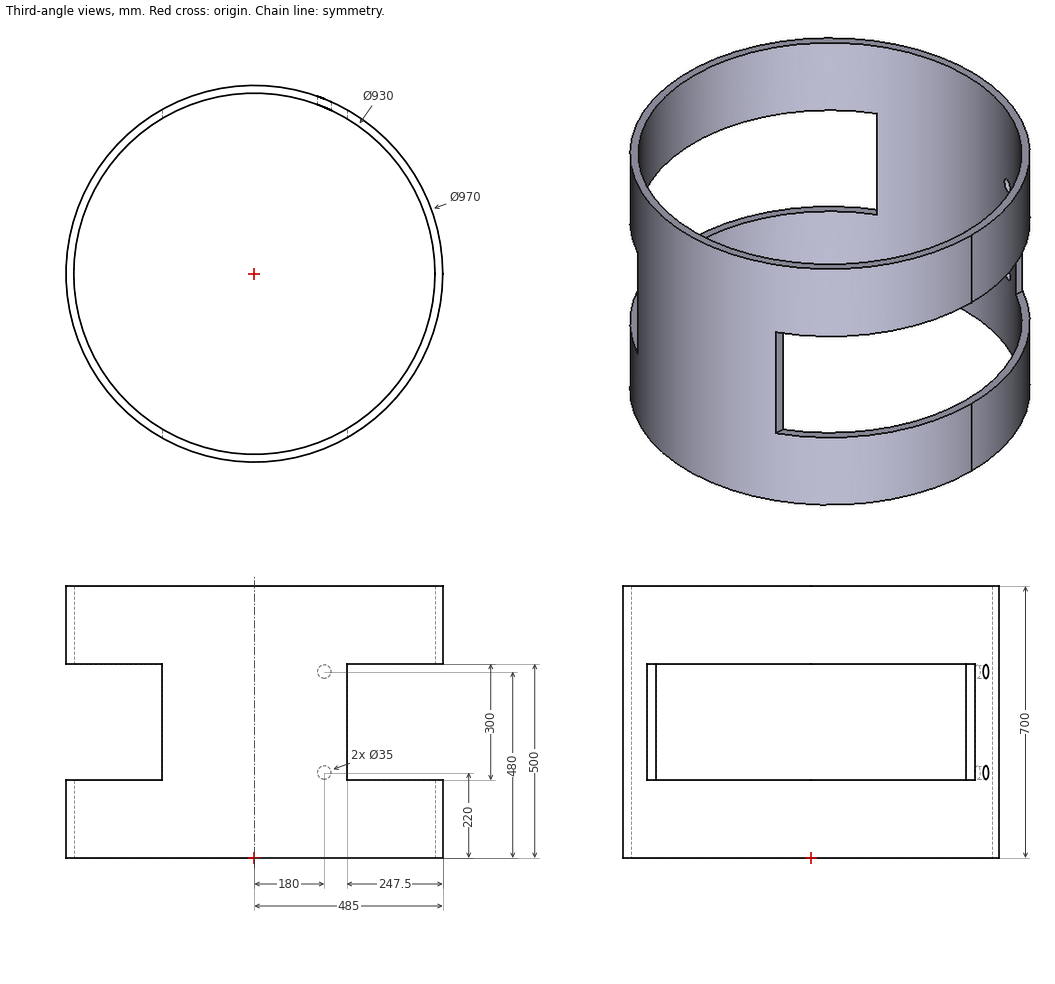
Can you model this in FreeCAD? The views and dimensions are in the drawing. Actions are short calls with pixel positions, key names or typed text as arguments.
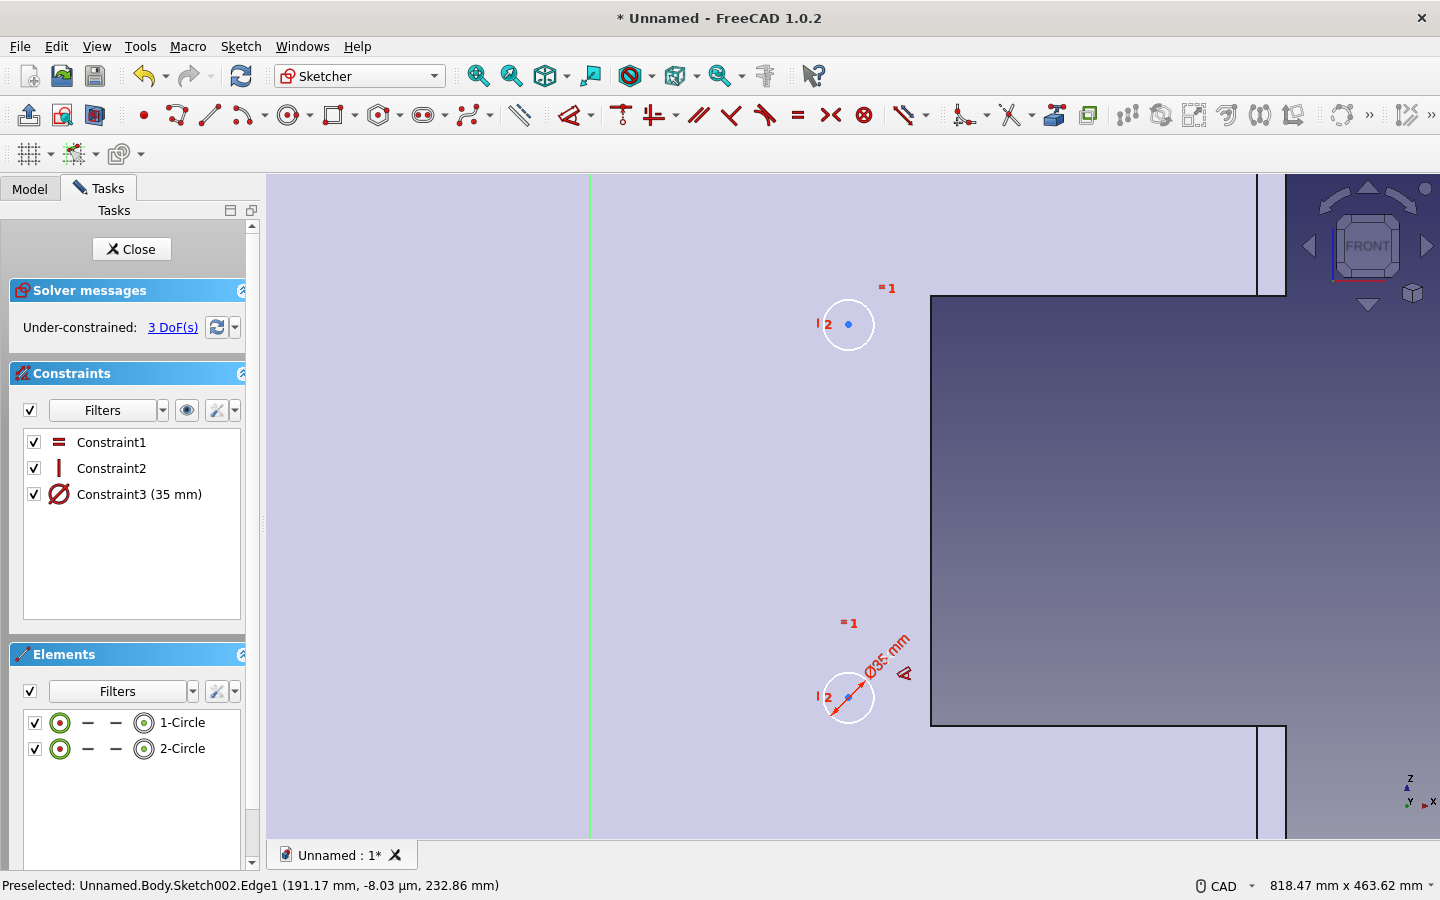
click(849, 698)
click(719, 664)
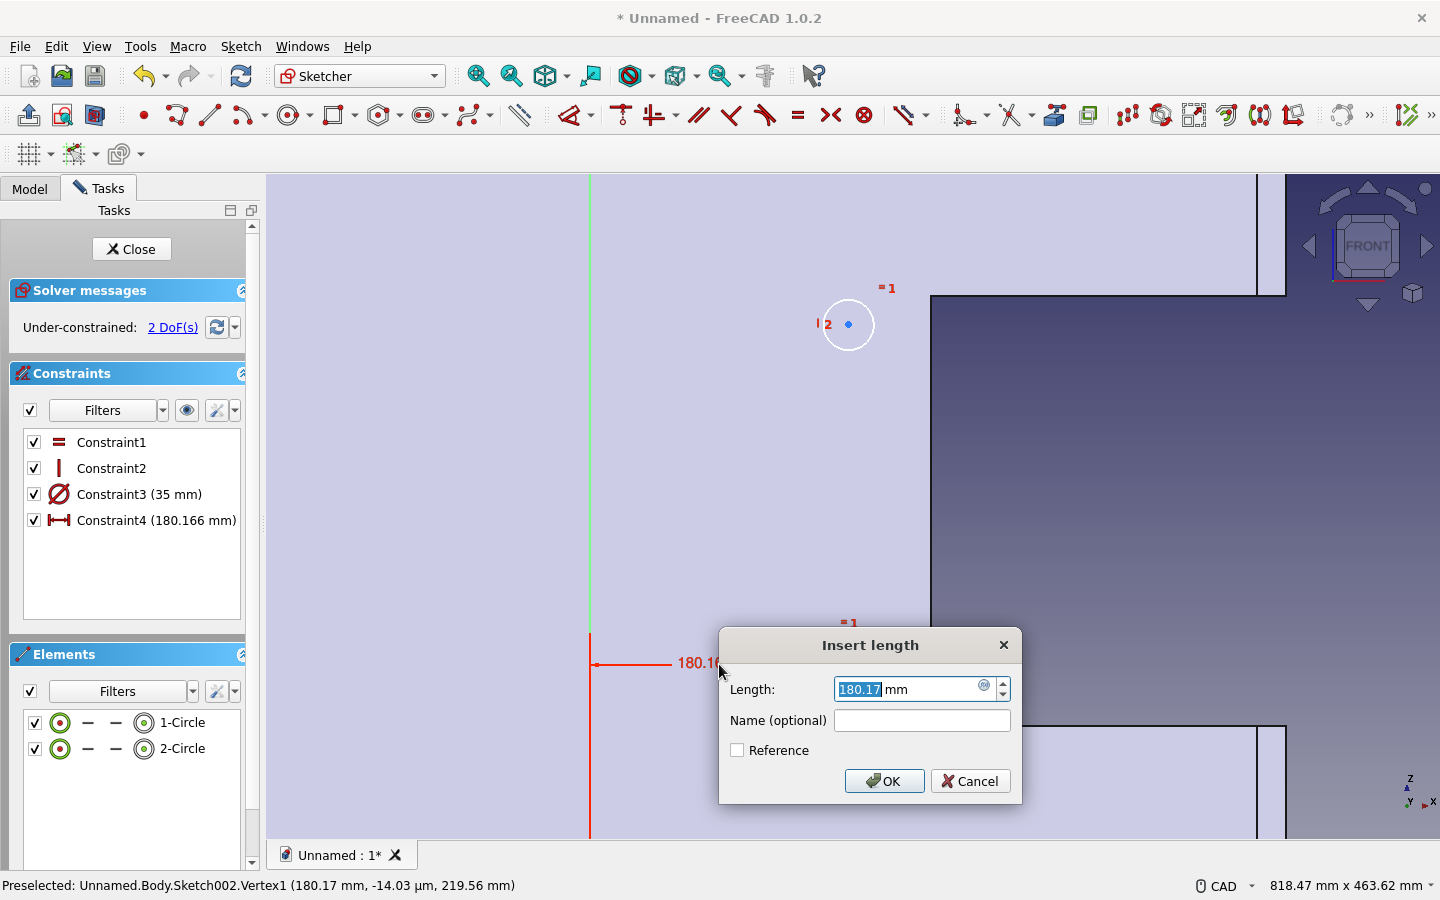
text(180)
key(Return)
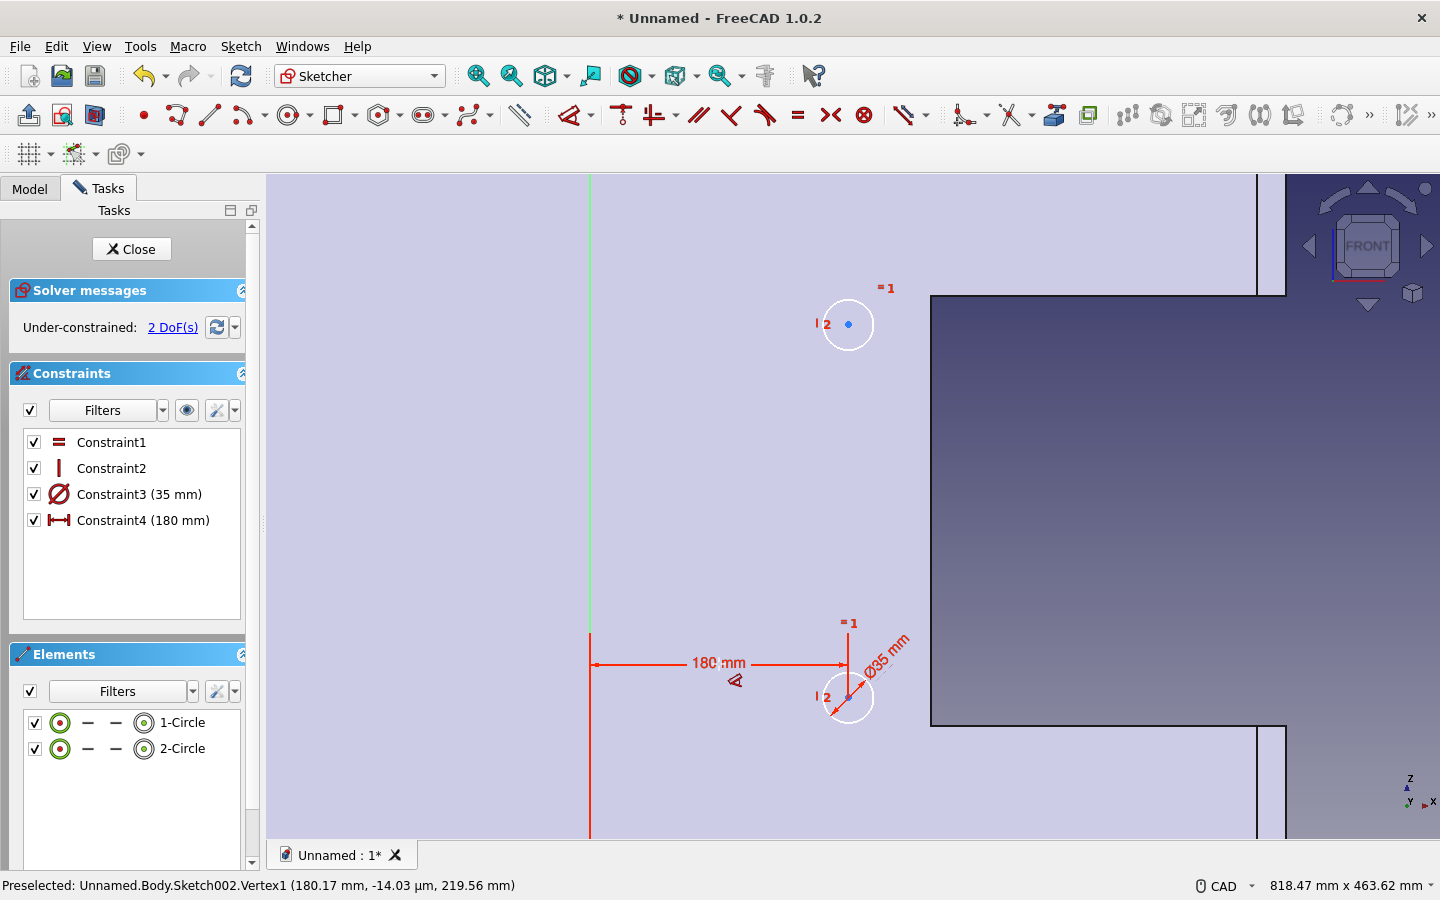
click(848, 698)
click(556, 754)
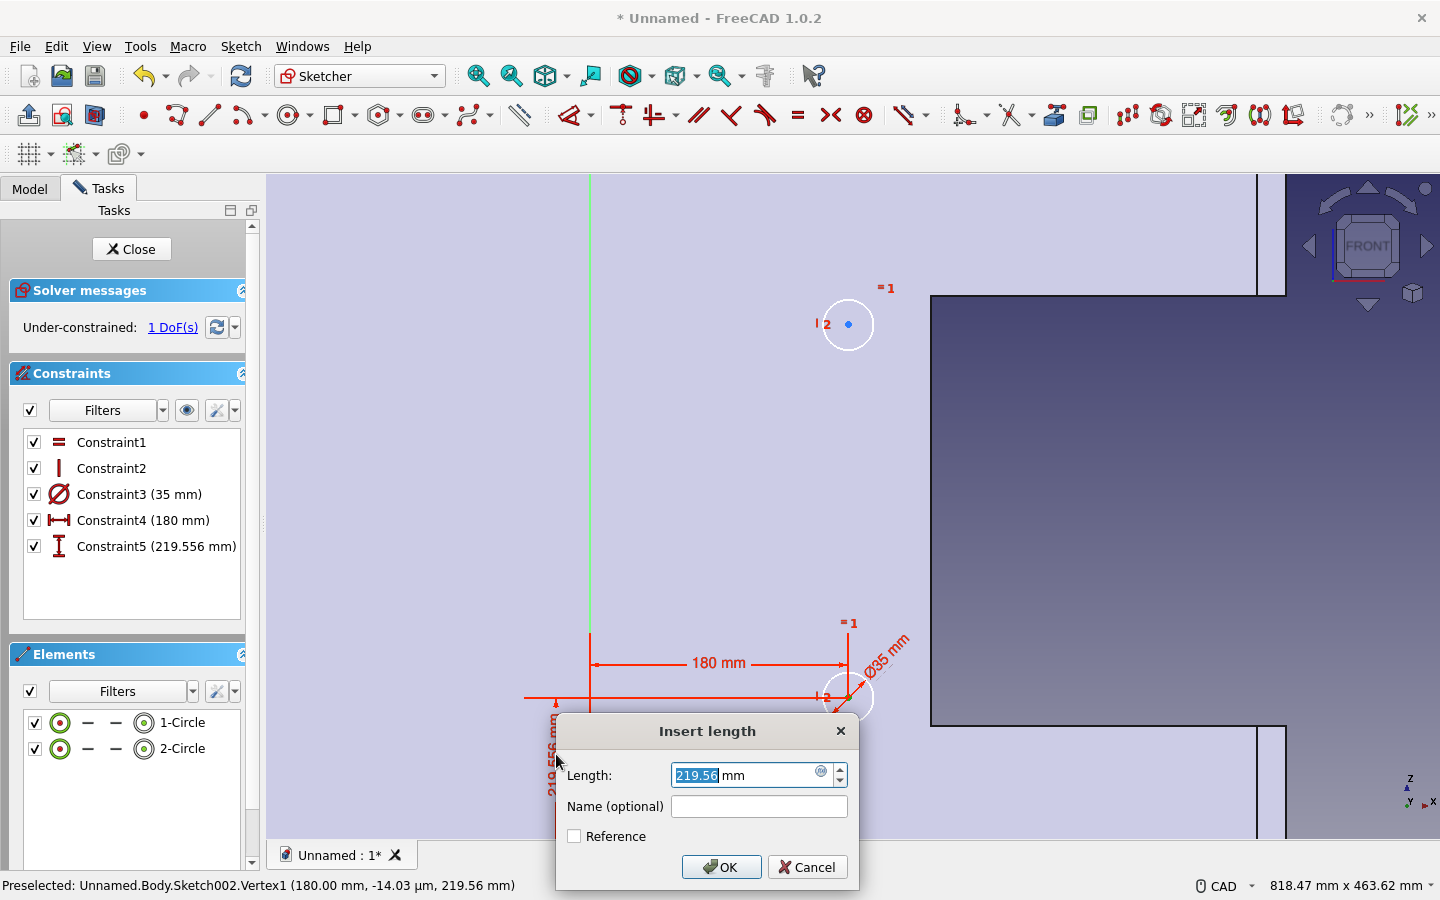
text(220)
key(Return)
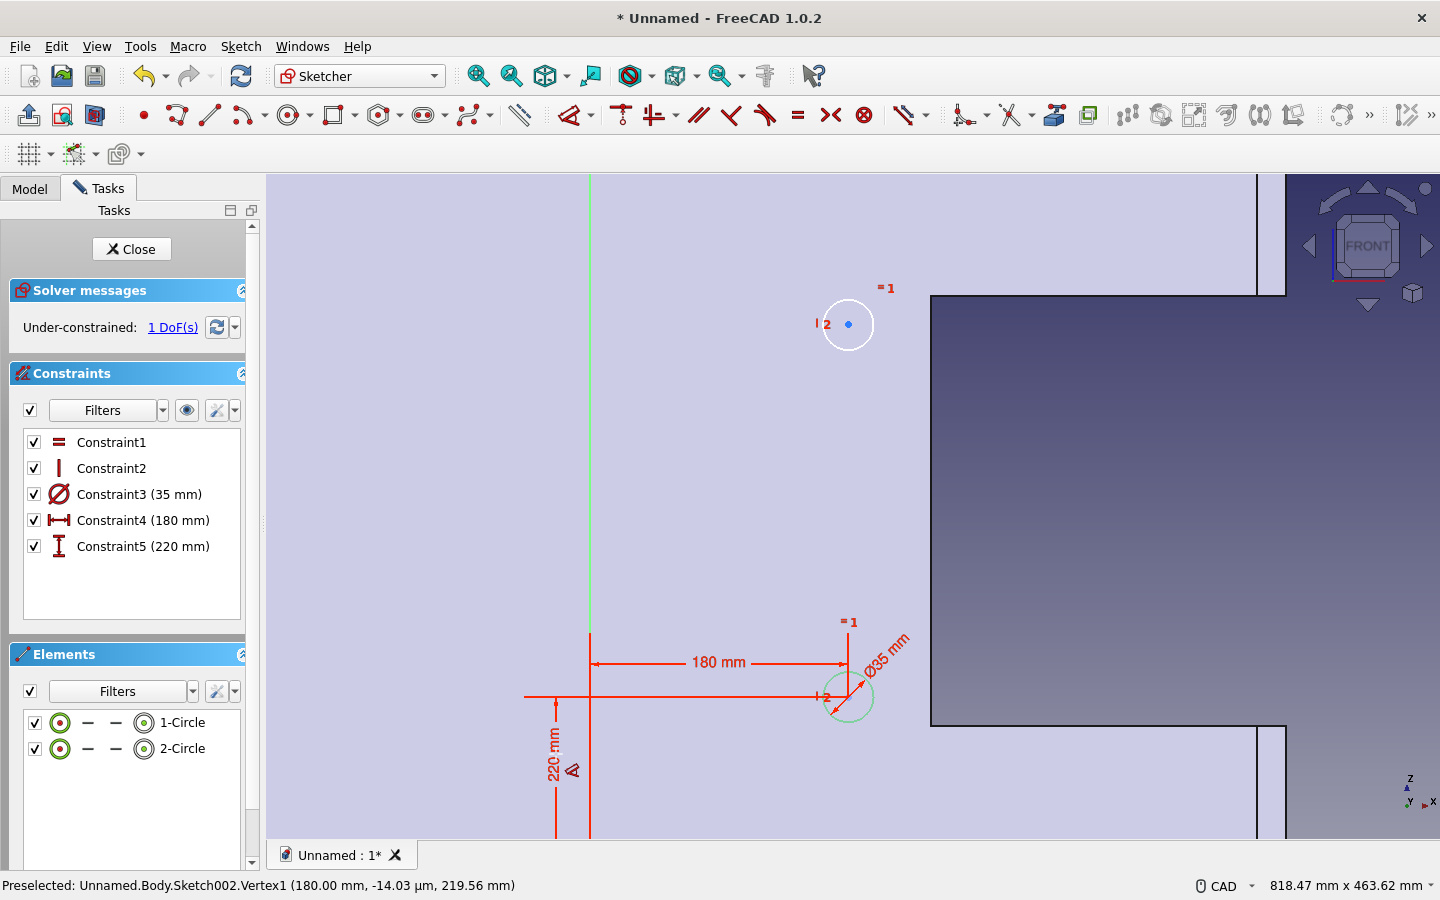
click(848, 325)
click(556, 568)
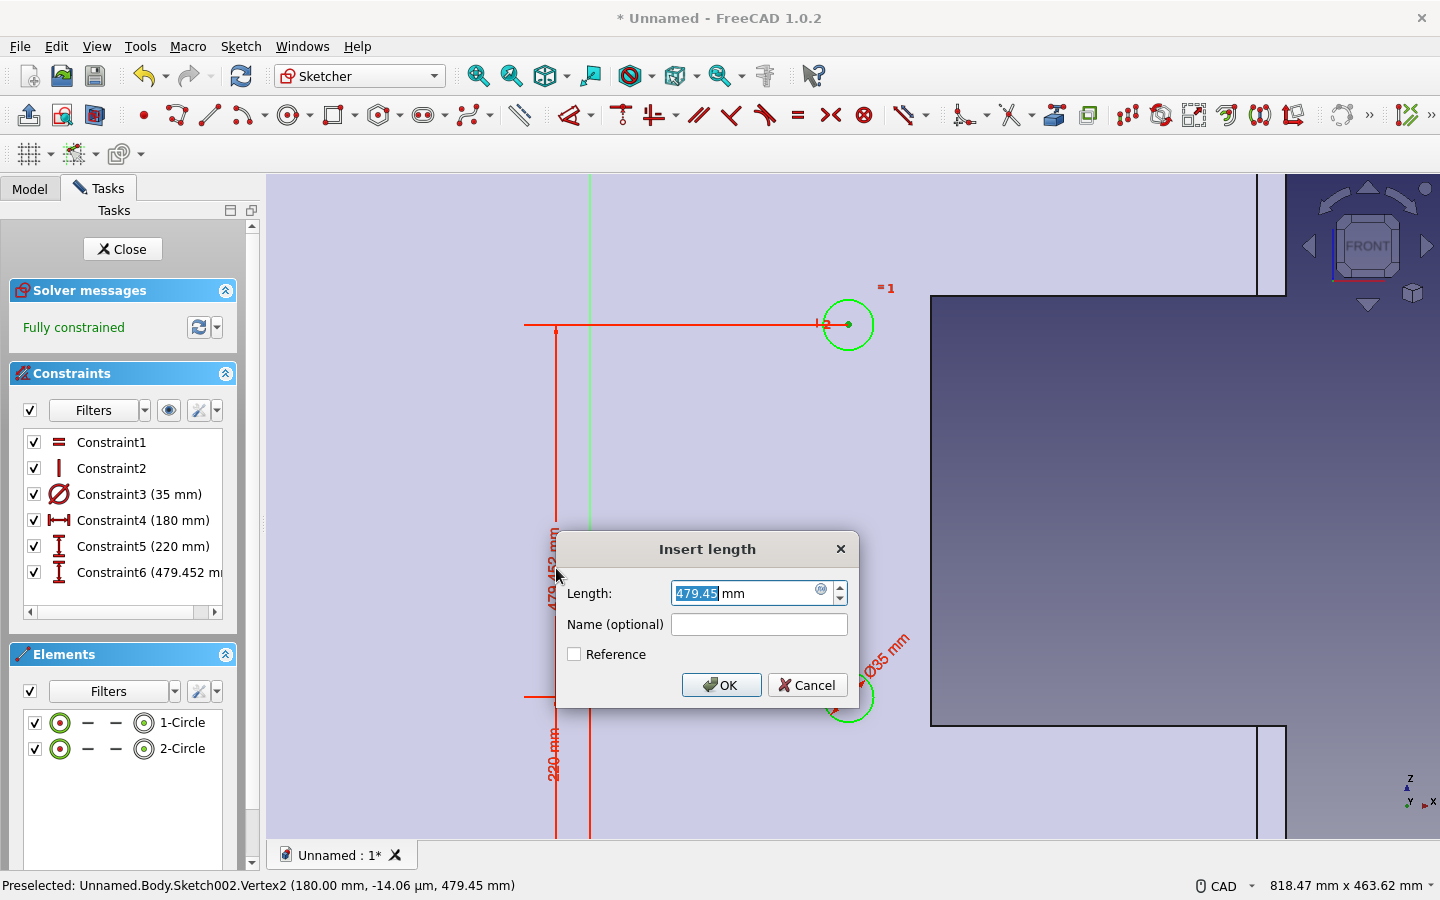
text(480)
key(Return)
key(Escape)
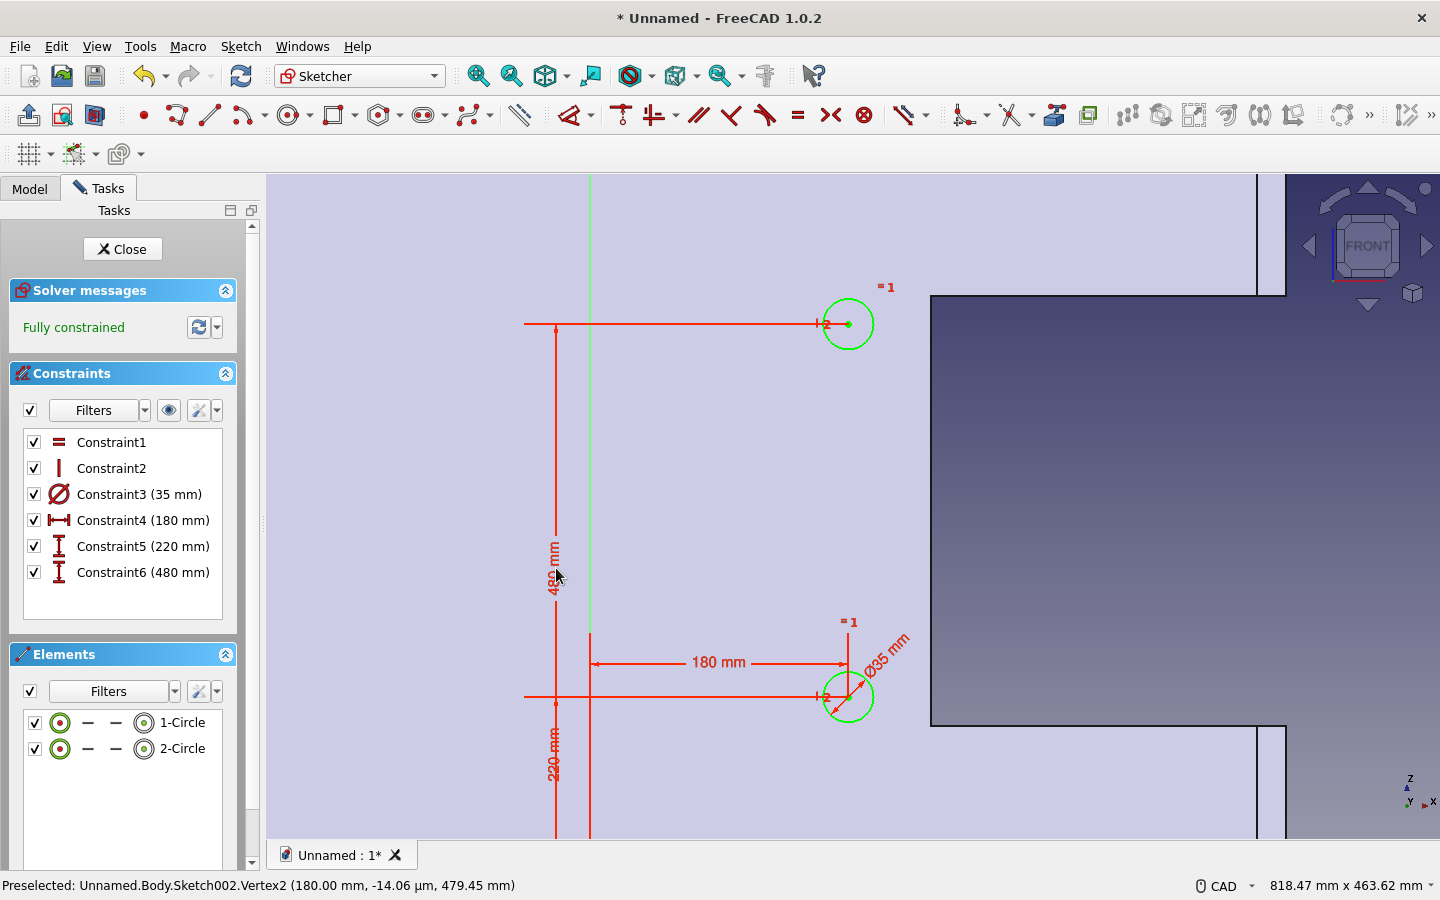
click(123, 249)